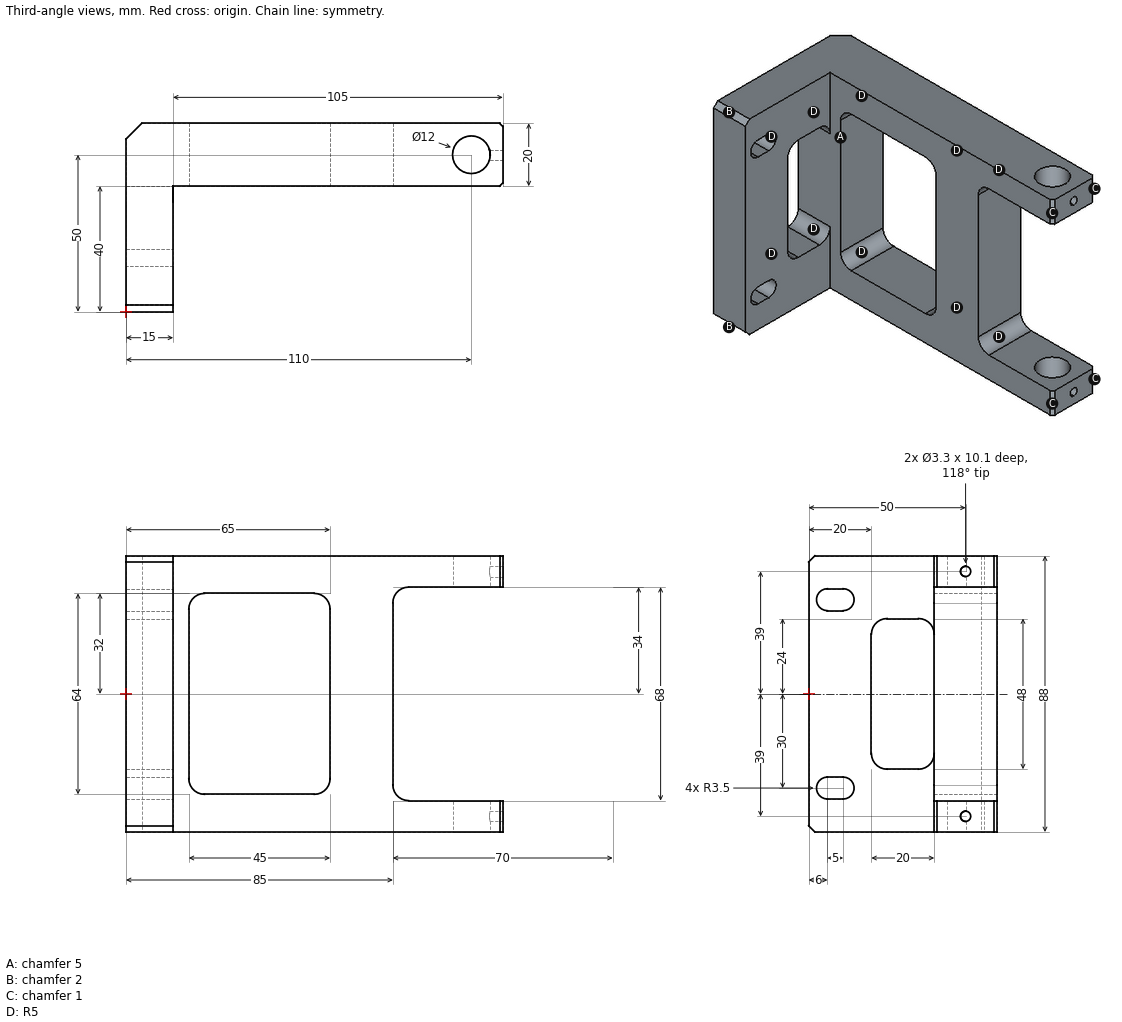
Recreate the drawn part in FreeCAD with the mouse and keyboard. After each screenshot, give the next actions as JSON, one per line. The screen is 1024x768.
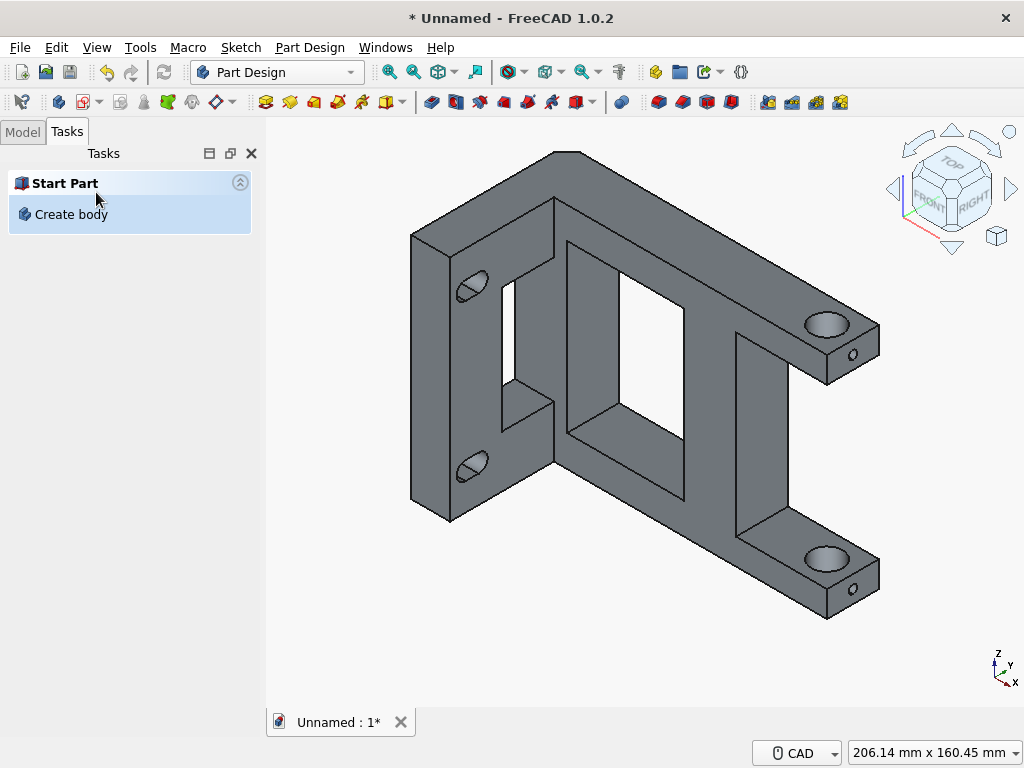
{"action": "left_click", "coordinate": [430, 245]}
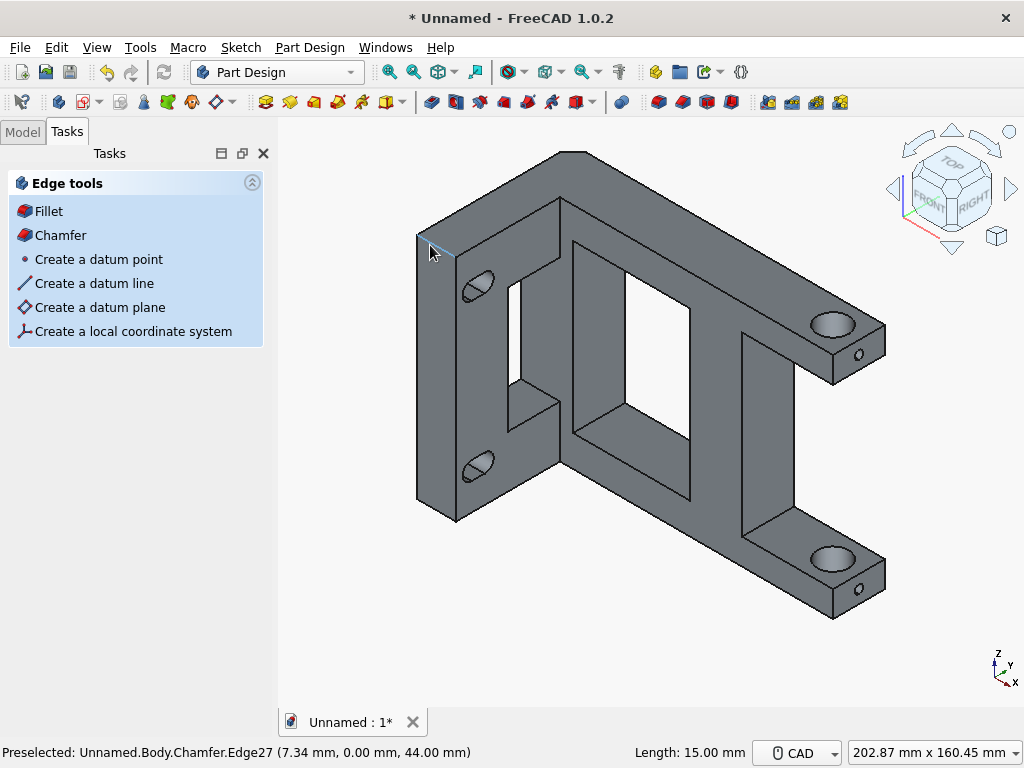
{"action": "key", "text": "2"}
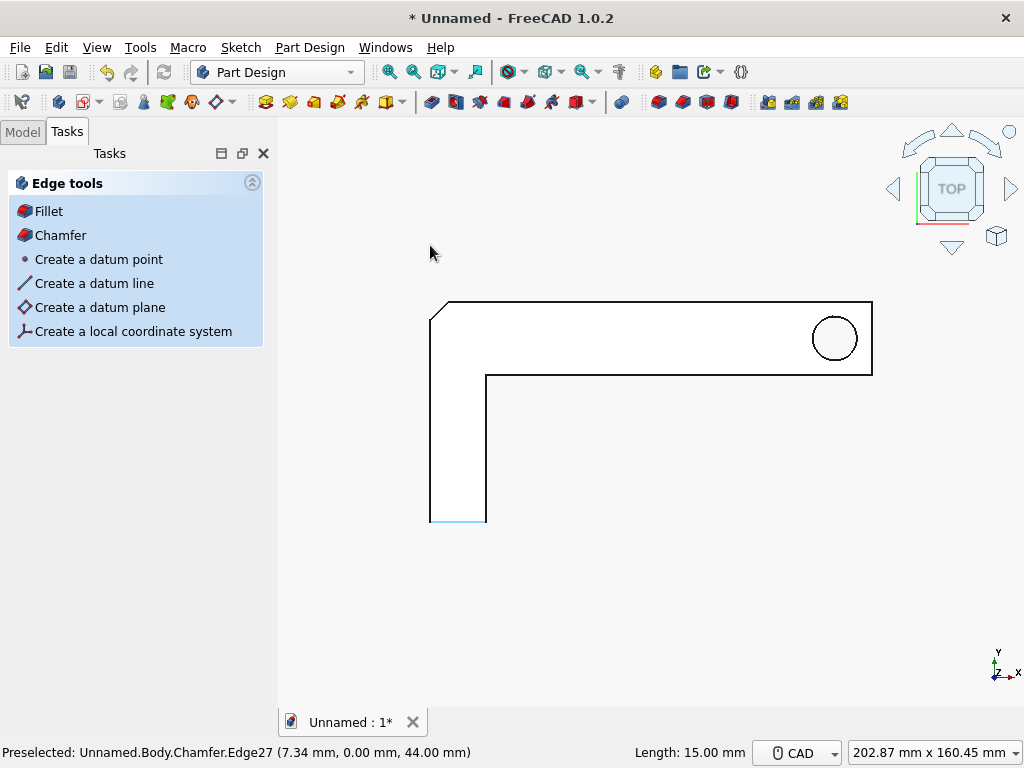
{"action": "key", "text": "1"}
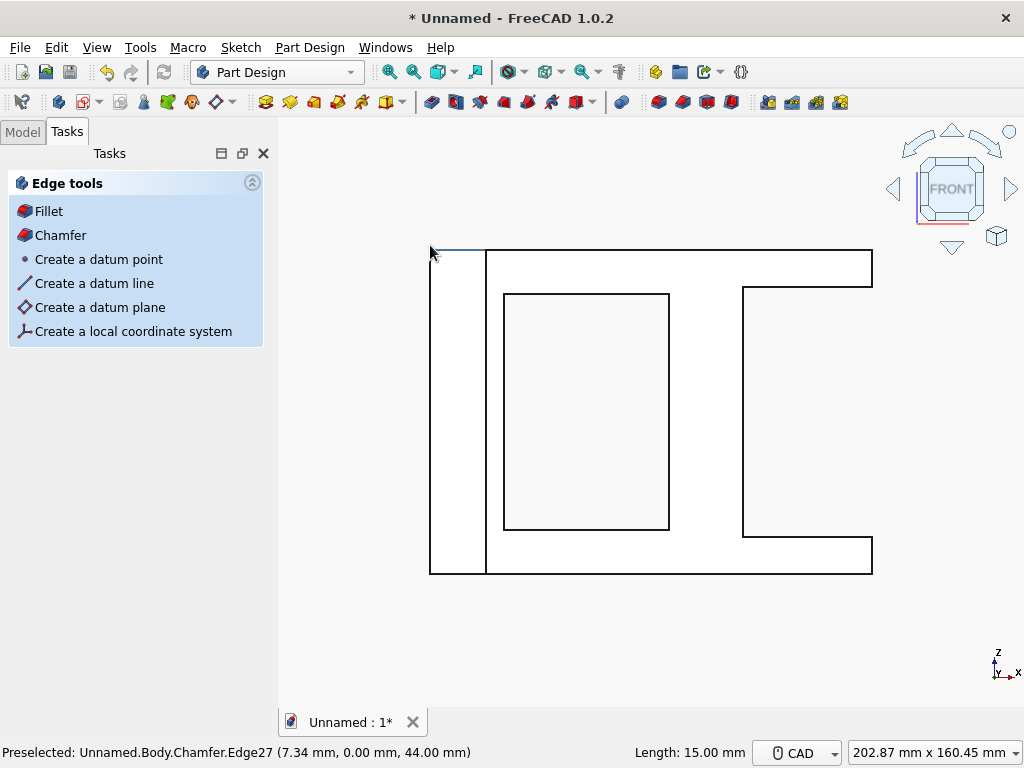
{"action": "left_click", "coordinate": [458, 573], "text": "ctrl"}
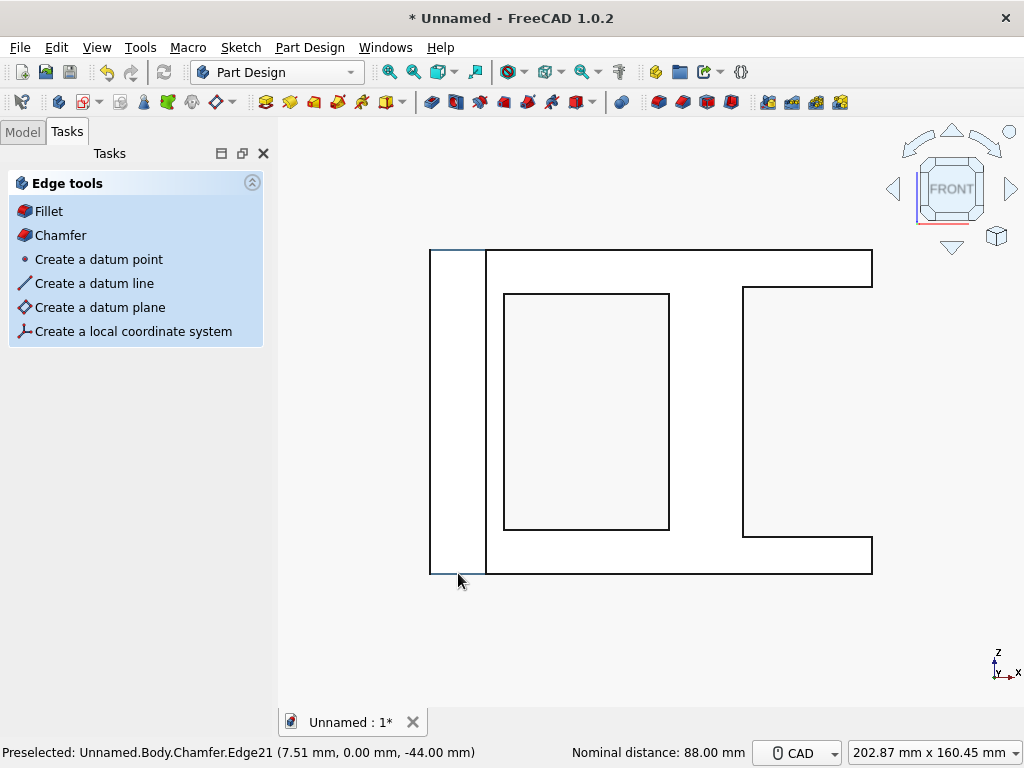
{"action": "left_click", "coordinate": [684, 102]}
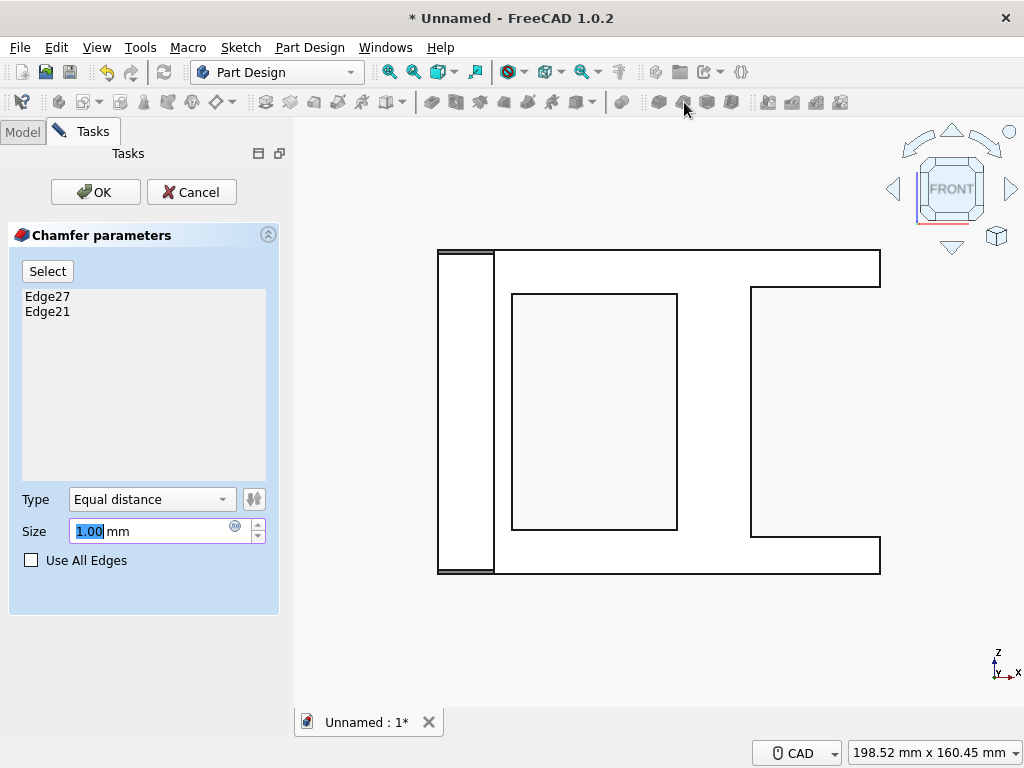
{"action": "type", "text": "2"}
{"action": "key", "text": "Tab"}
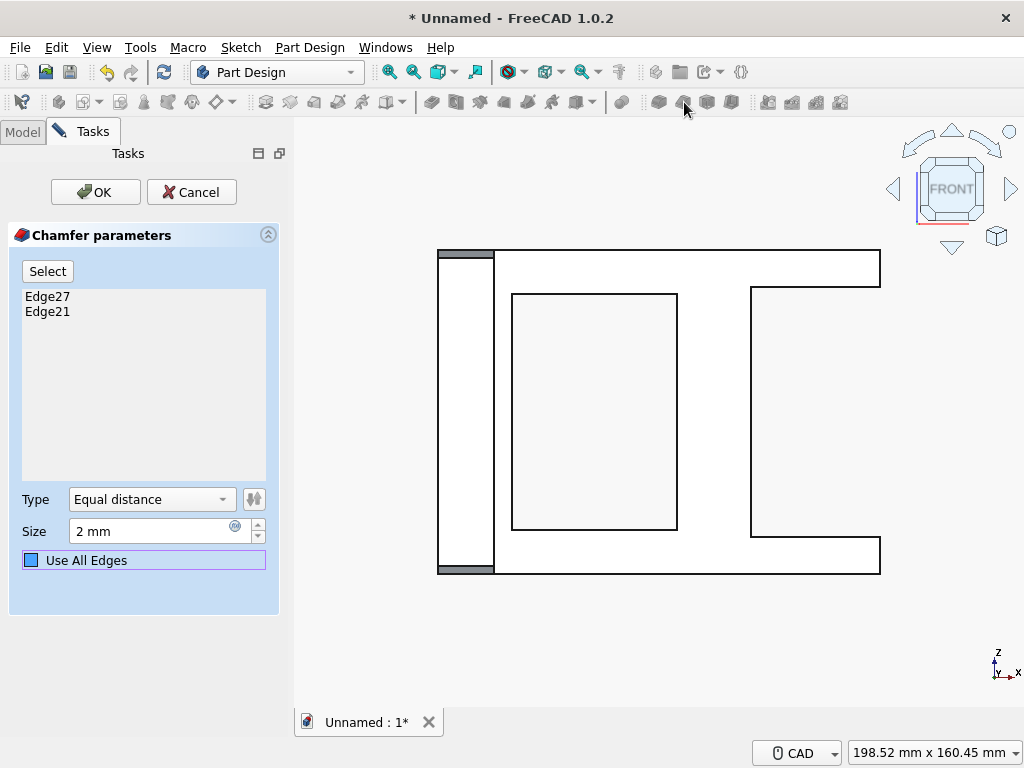
{"action": "left_click", "coordinate": [96, 192]}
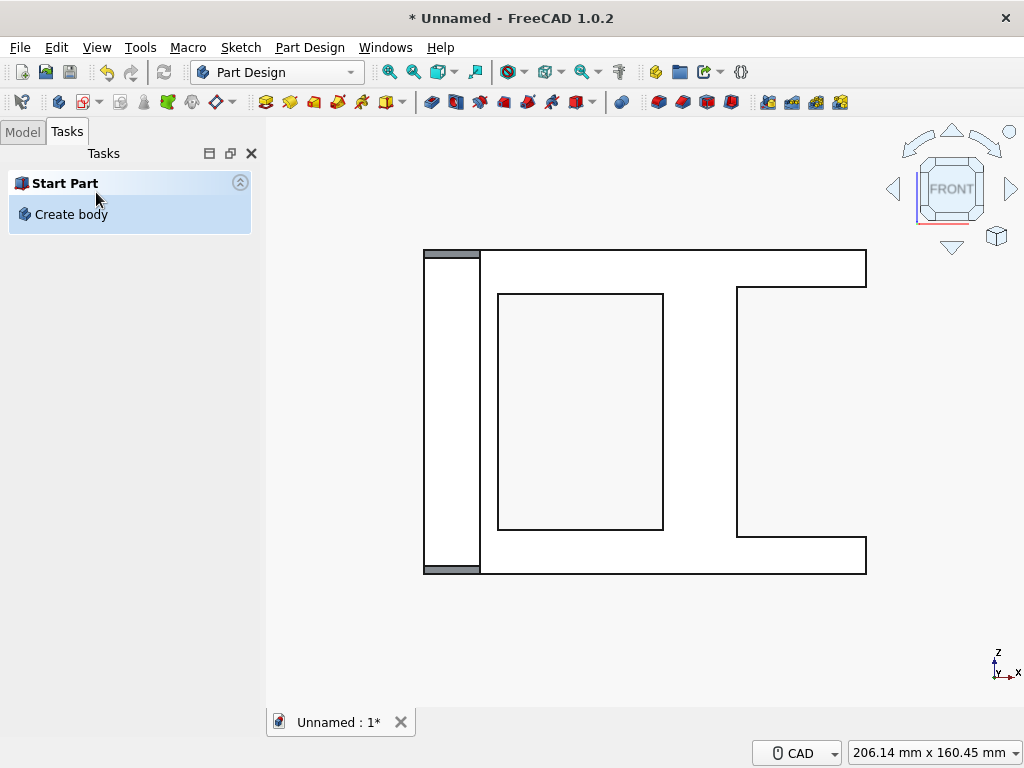
{"action": "left_click", "coordinate": [866, 554]}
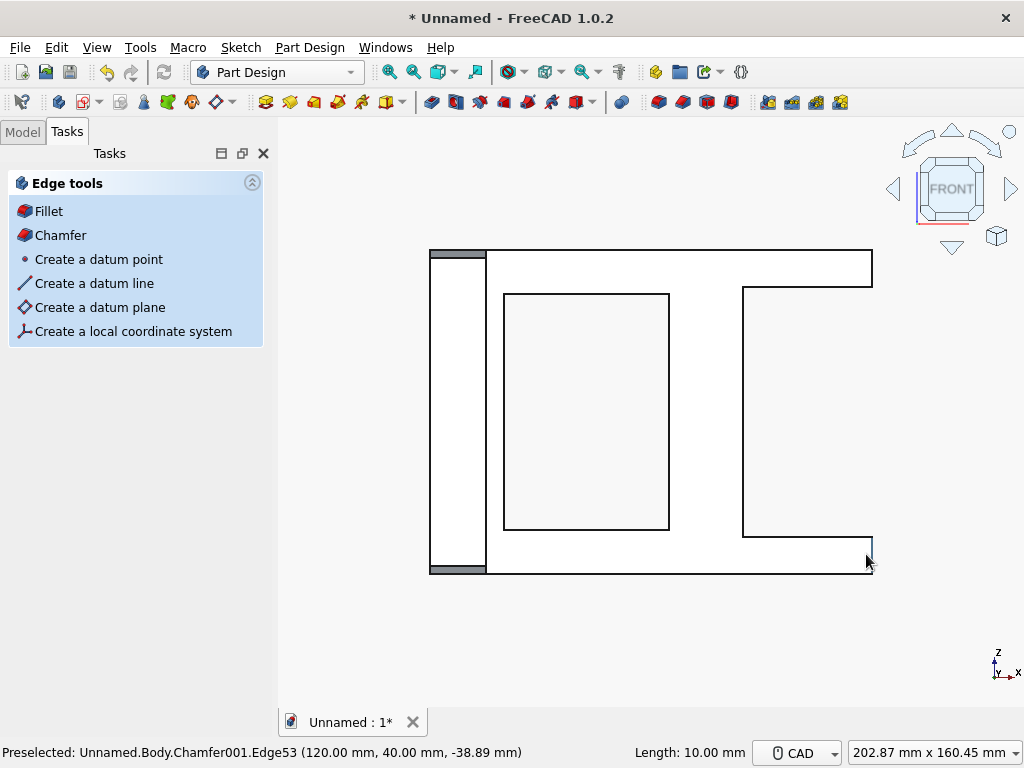
{"action": "key", "text": "0"}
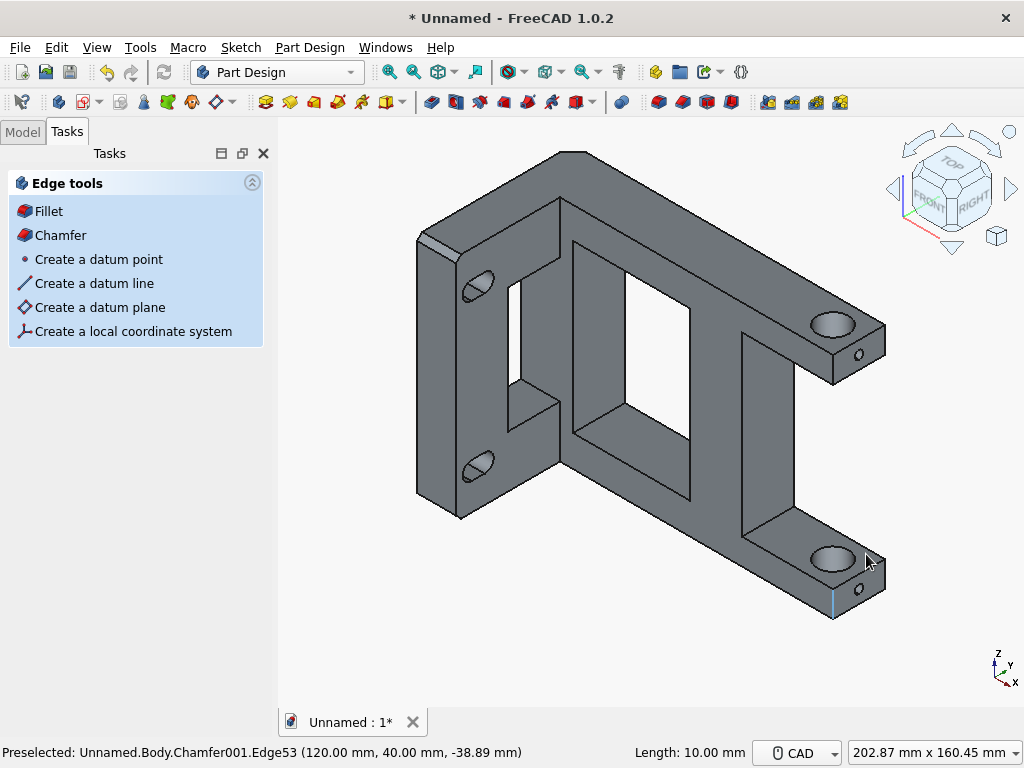
{"action": "left_click", "coordinate": [833, 369], "text": "ctrl"}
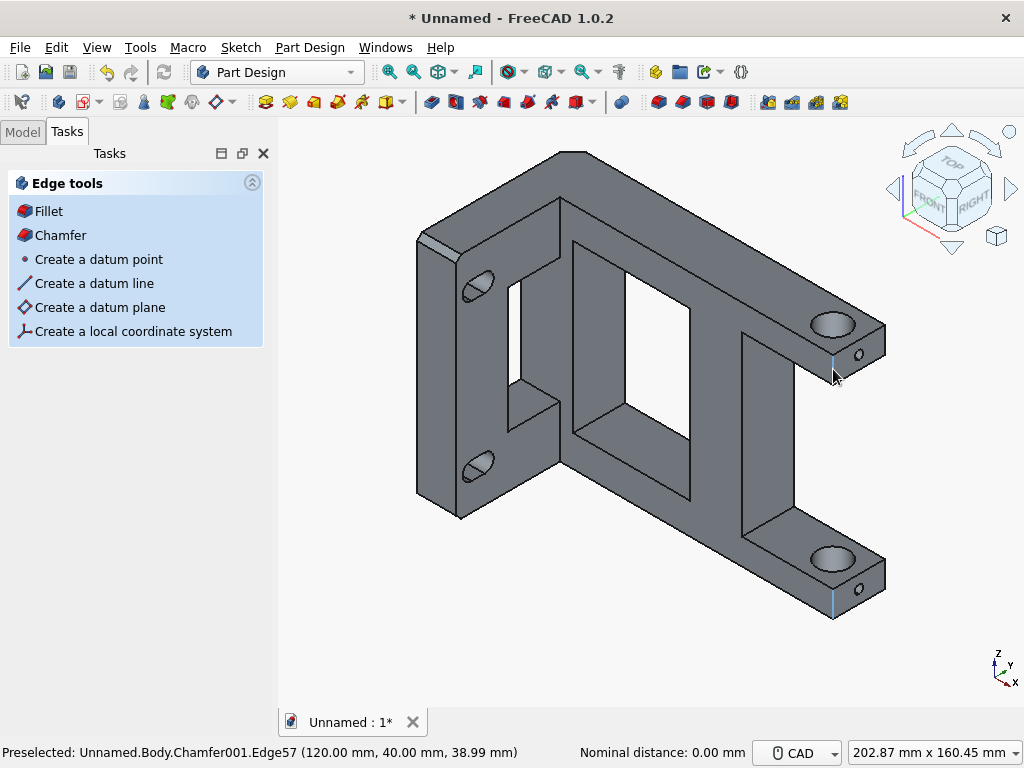
{"action": "key", "text": "2"}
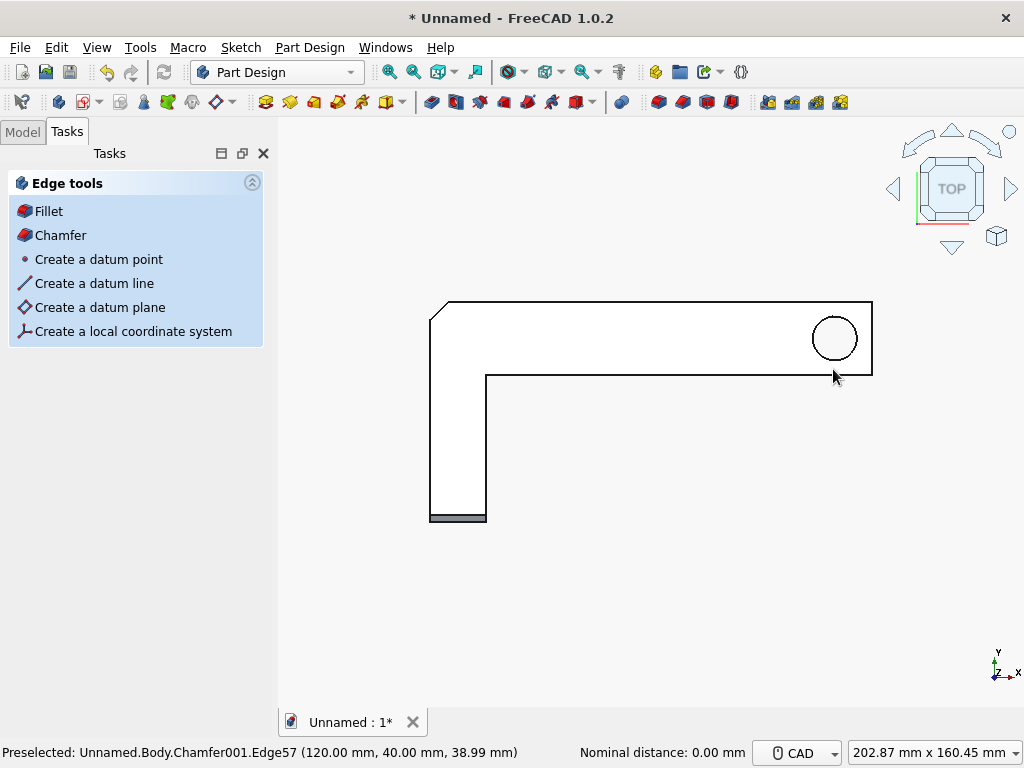
{"action": "key", "text": "1"}